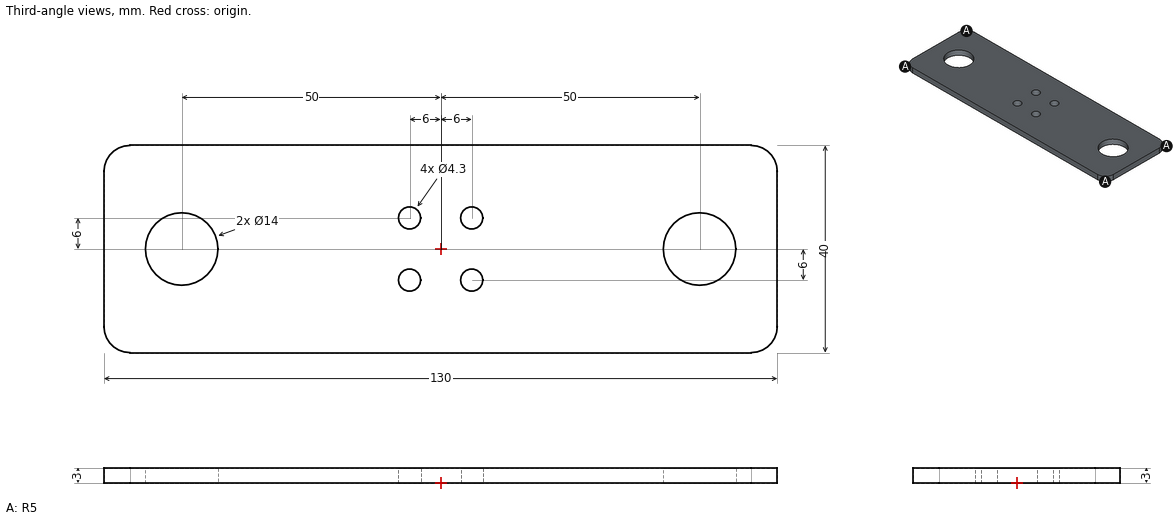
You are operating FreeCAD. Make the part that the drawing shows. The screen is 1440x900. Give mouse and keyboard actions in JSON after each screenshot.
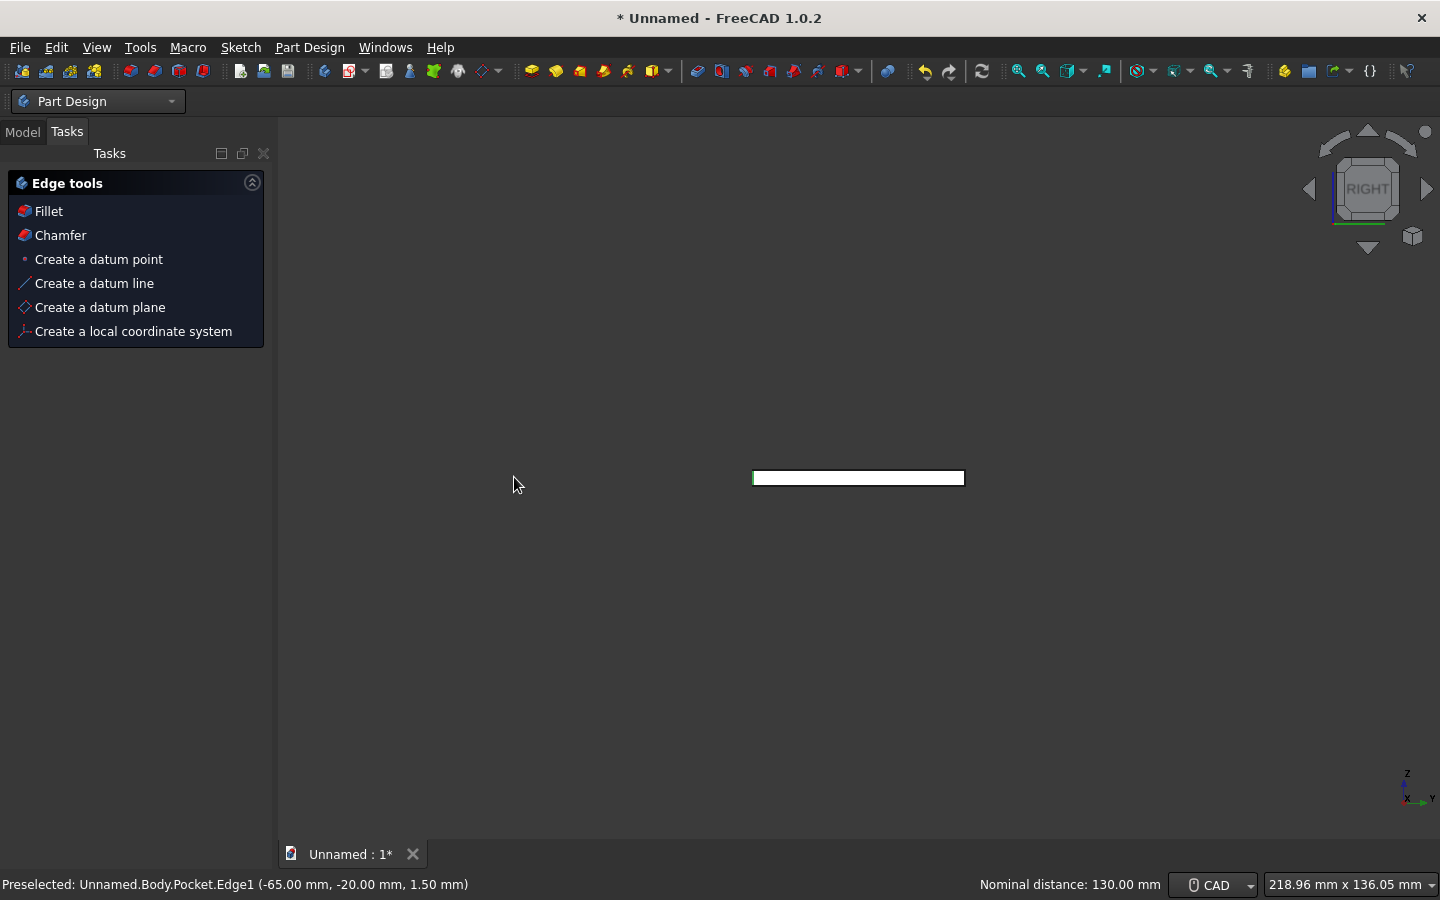
{"action": "left_click", "coordinate": [1020, 72]}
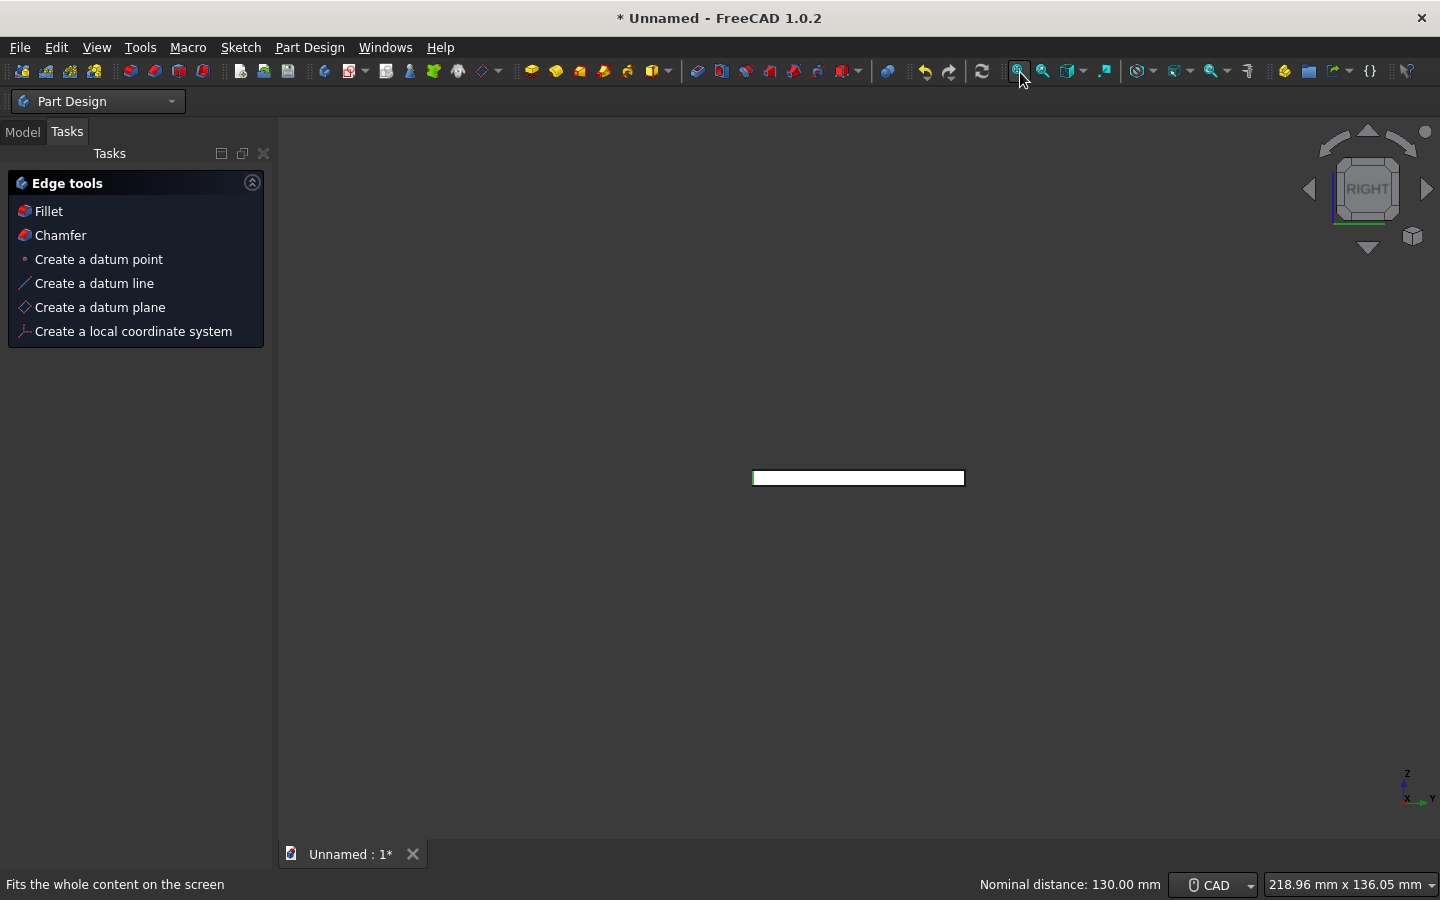
{"action": "left_click", "coordinate": [965, 477], "text": "ctrl"}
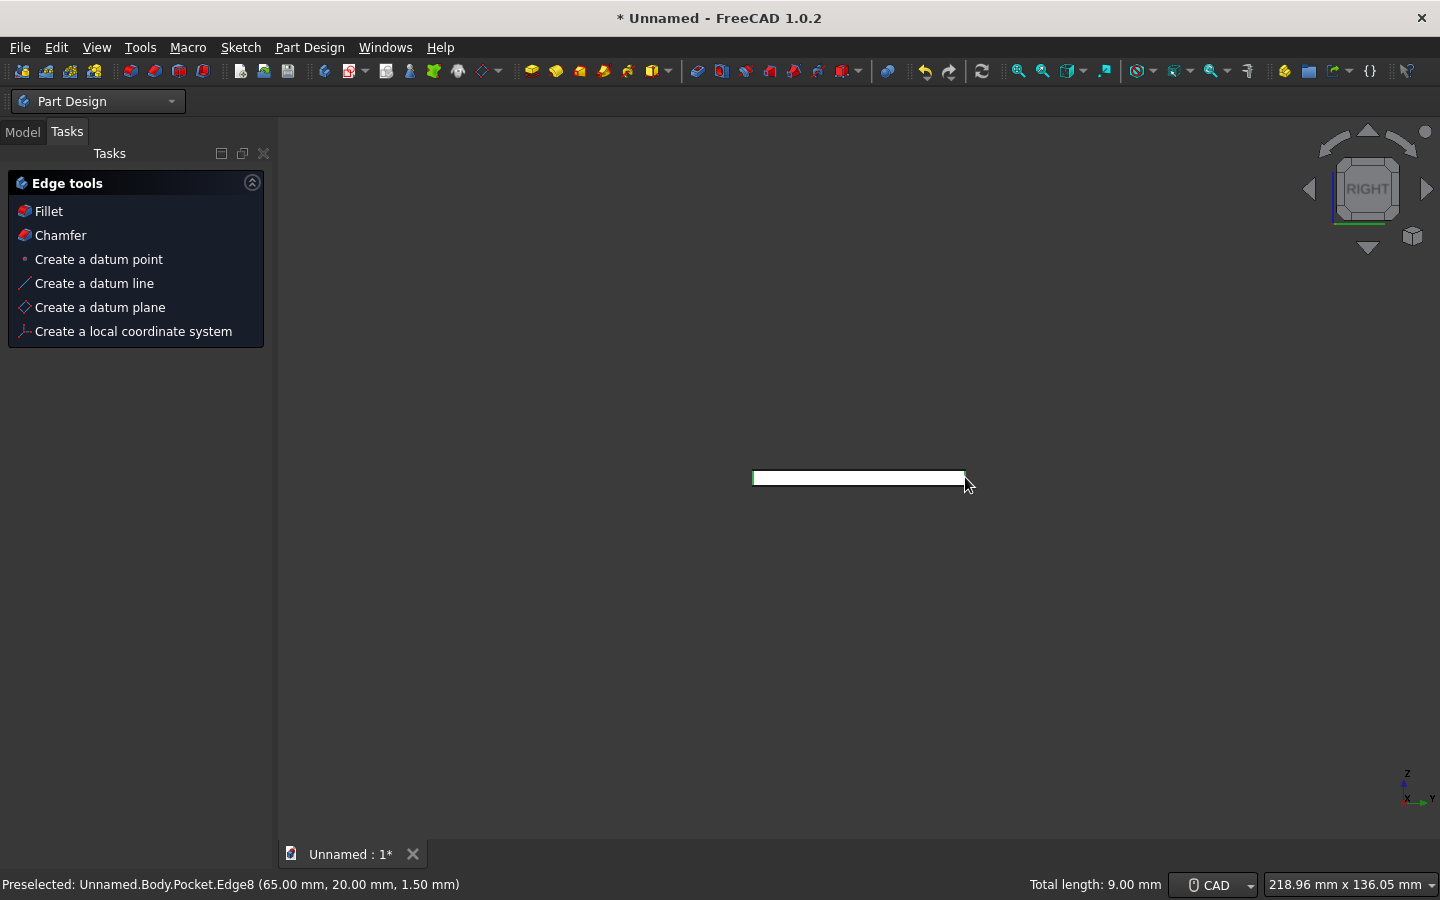
{"action": "scroll", "coordinate": [965, 477], "scroll_direction": "up", "scroll_amount": 5}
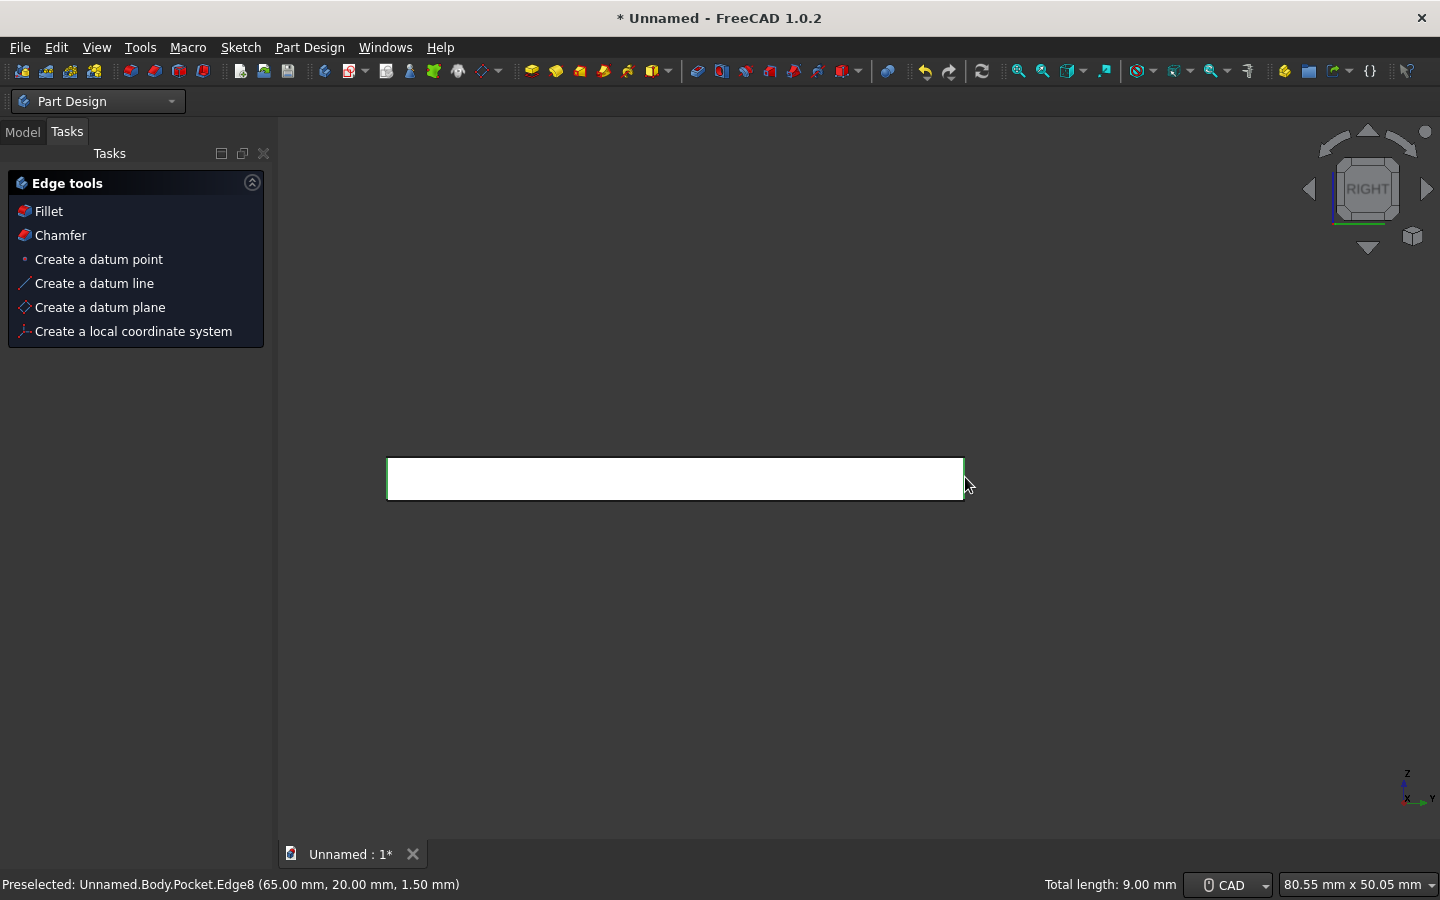
{"action": "key", "text": "v f"}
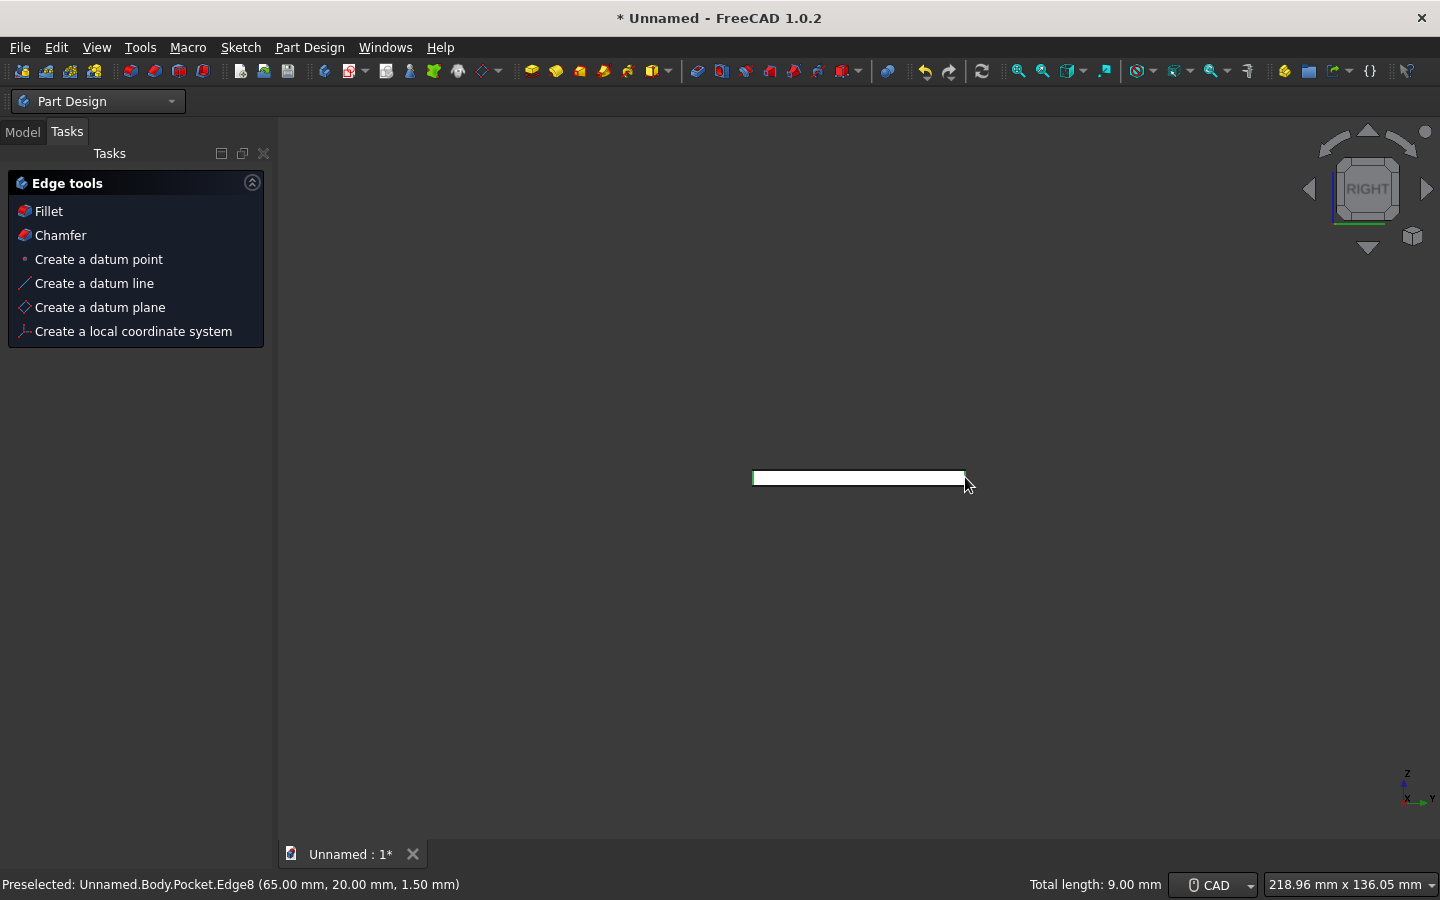
{"action": "key", "text": "5"}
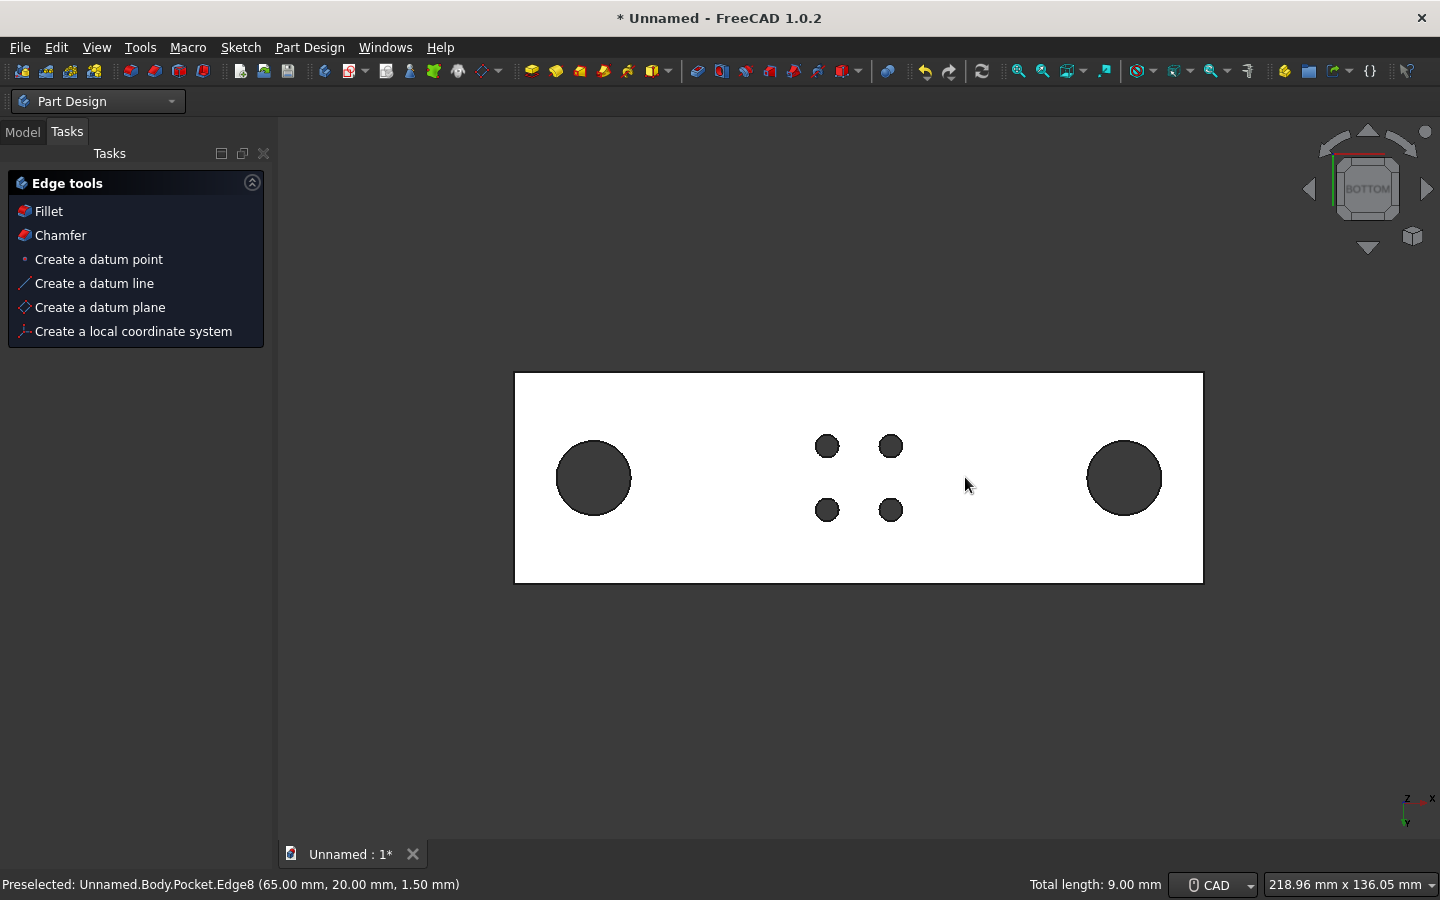
{"action": "scroll", "coordinate": [514, 583], "scroll_direction": "up", "scroll_amount": 5}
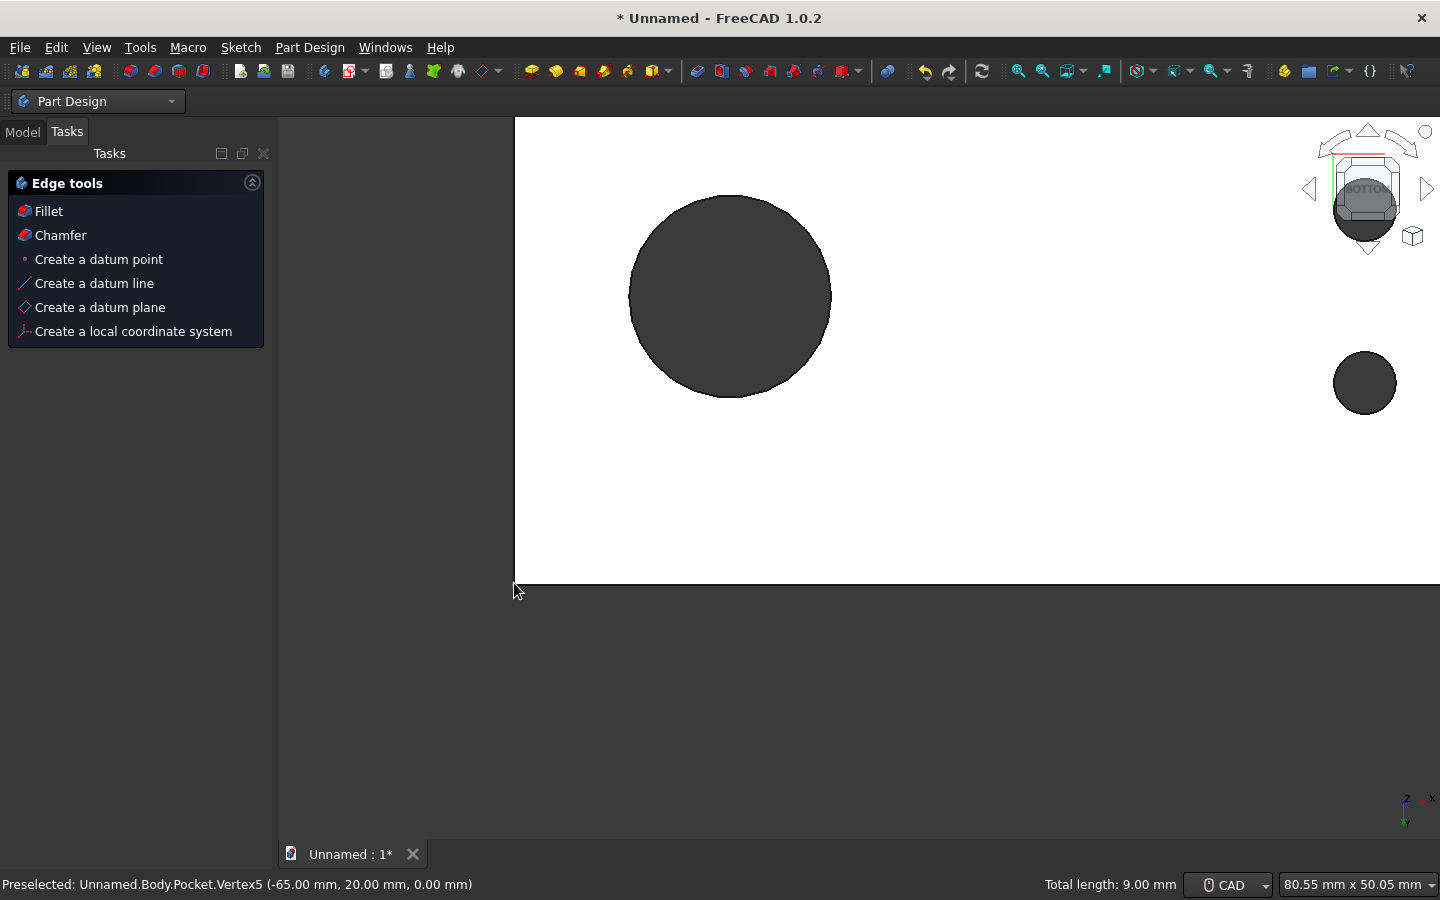
{"action": "key", "text": "v f"}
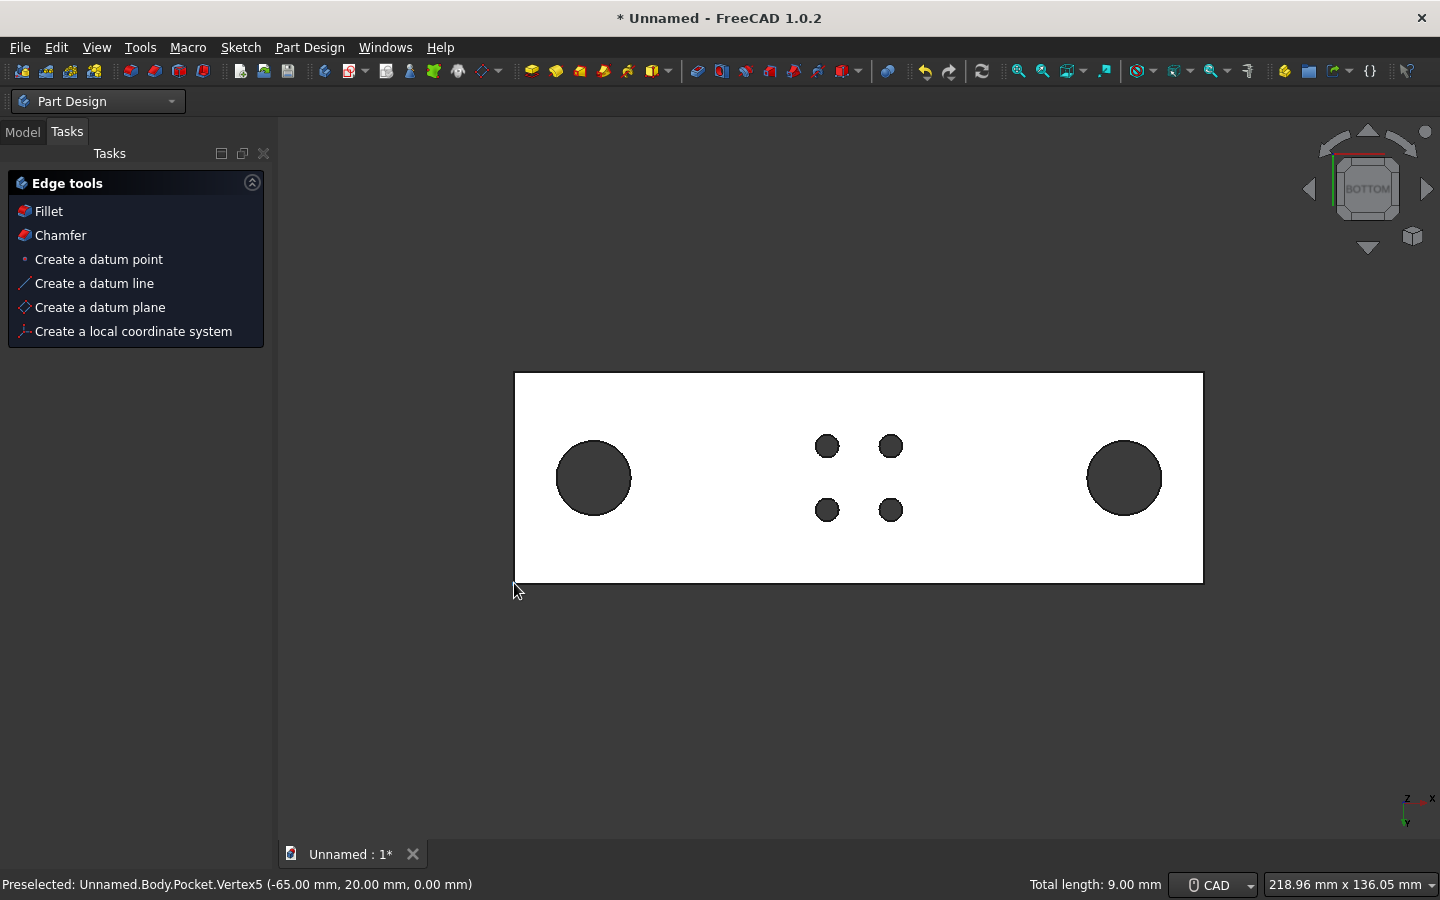
{"action": "key", "text": "4"}